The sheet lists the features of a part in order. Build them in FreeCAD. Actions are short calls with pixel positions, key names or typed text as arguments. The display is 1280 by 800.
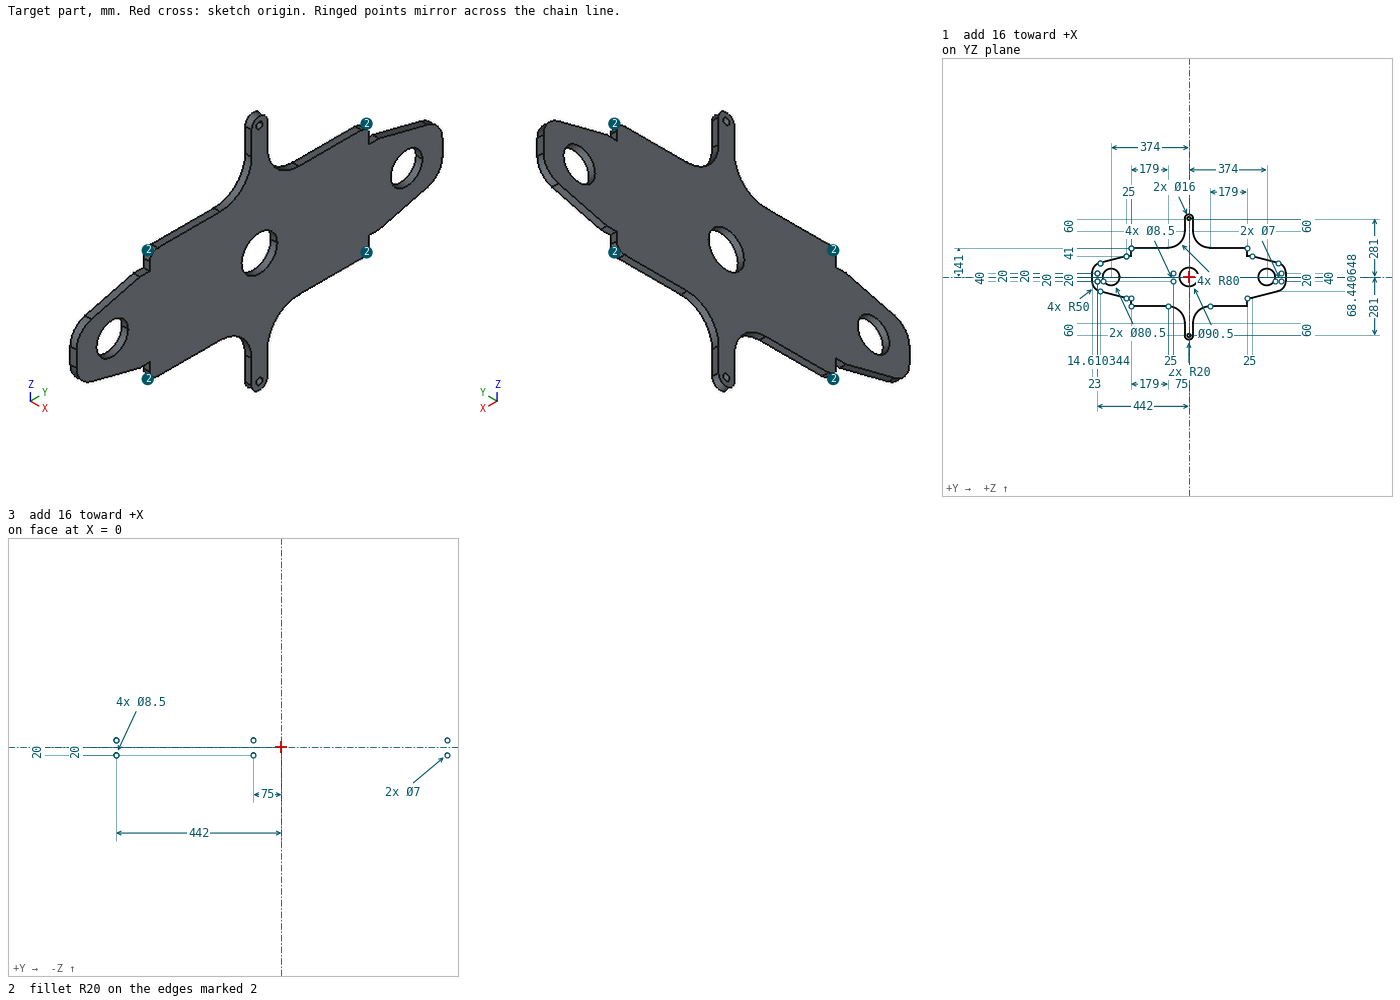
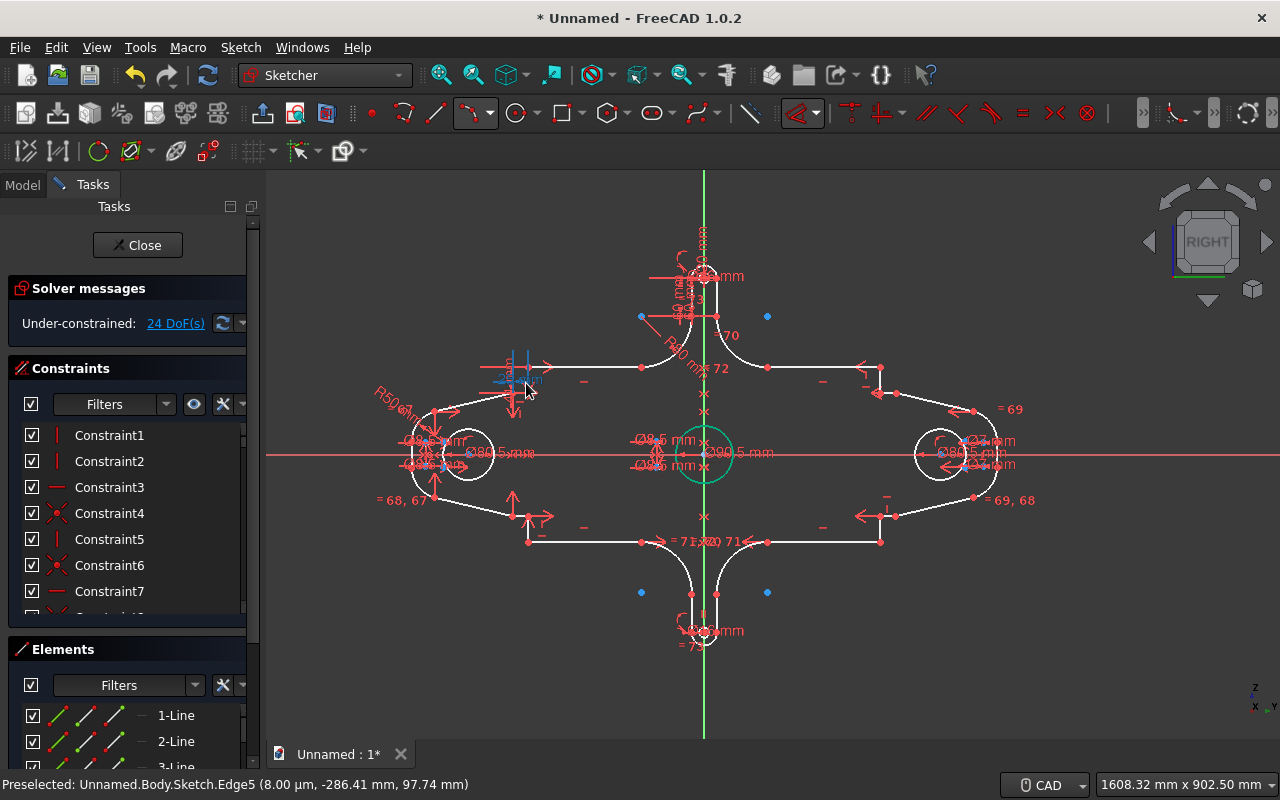
scroll(412, 450, up, 6)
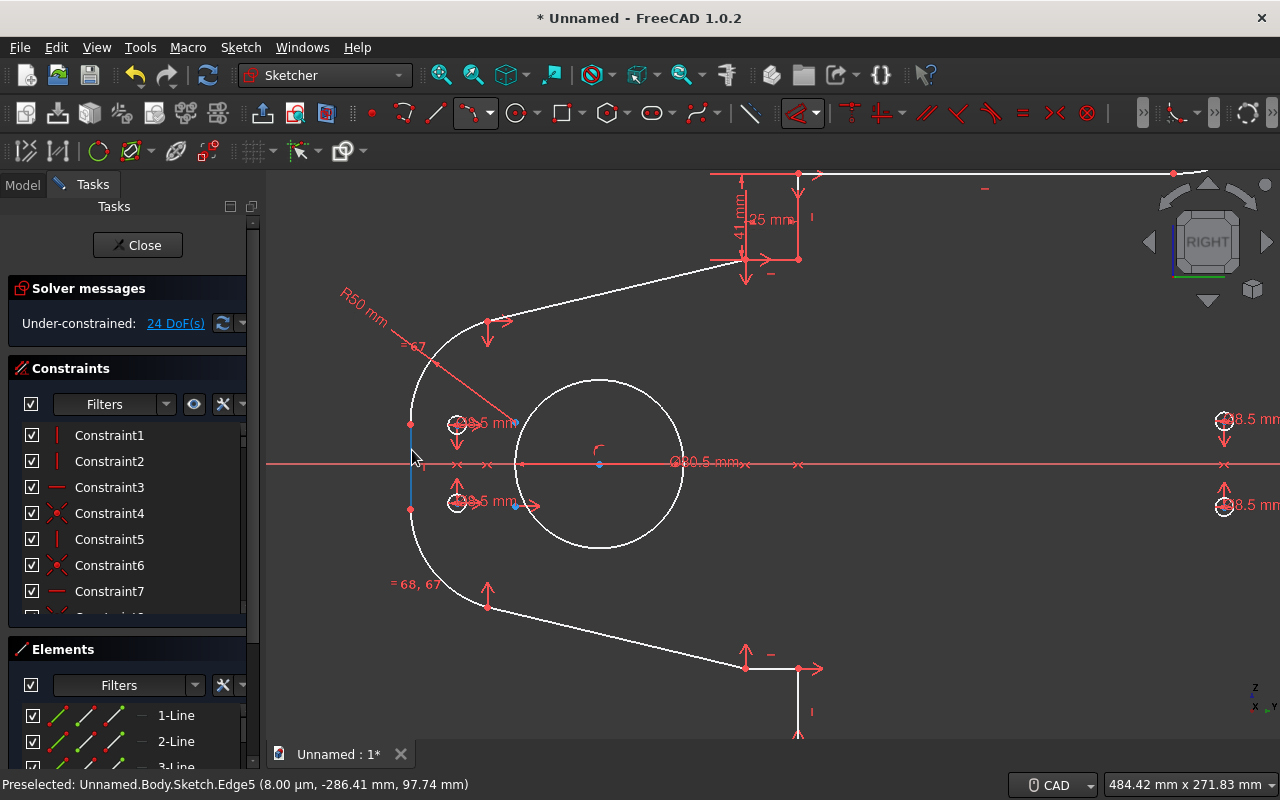
click(411, 450)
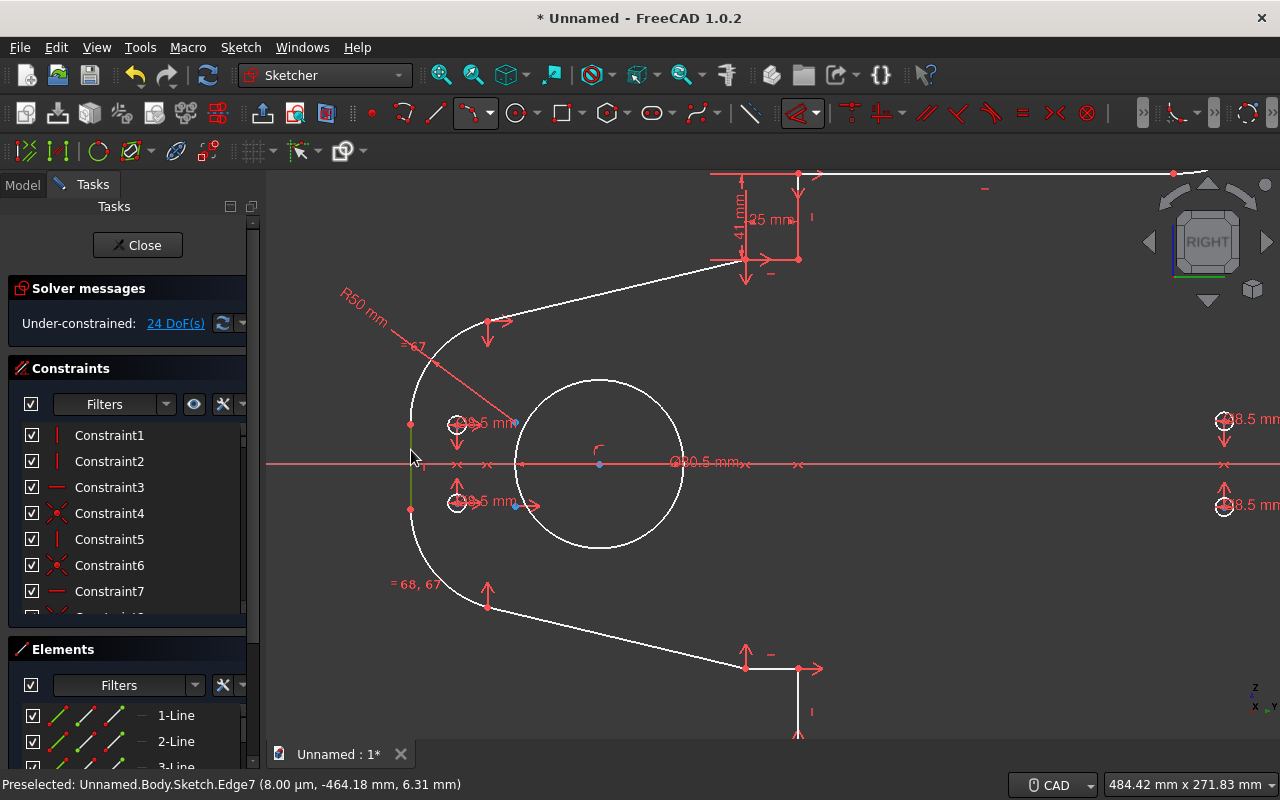
key(i)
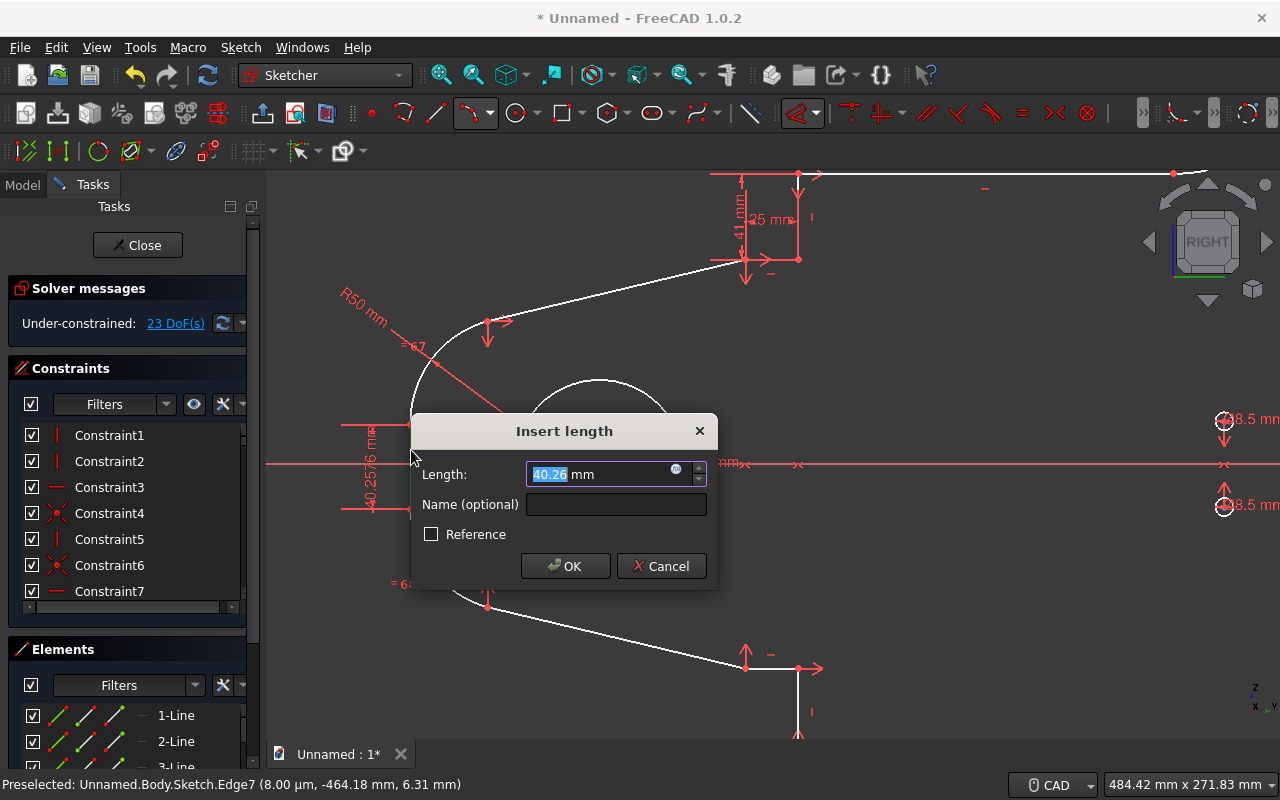
text(40)
key(Return)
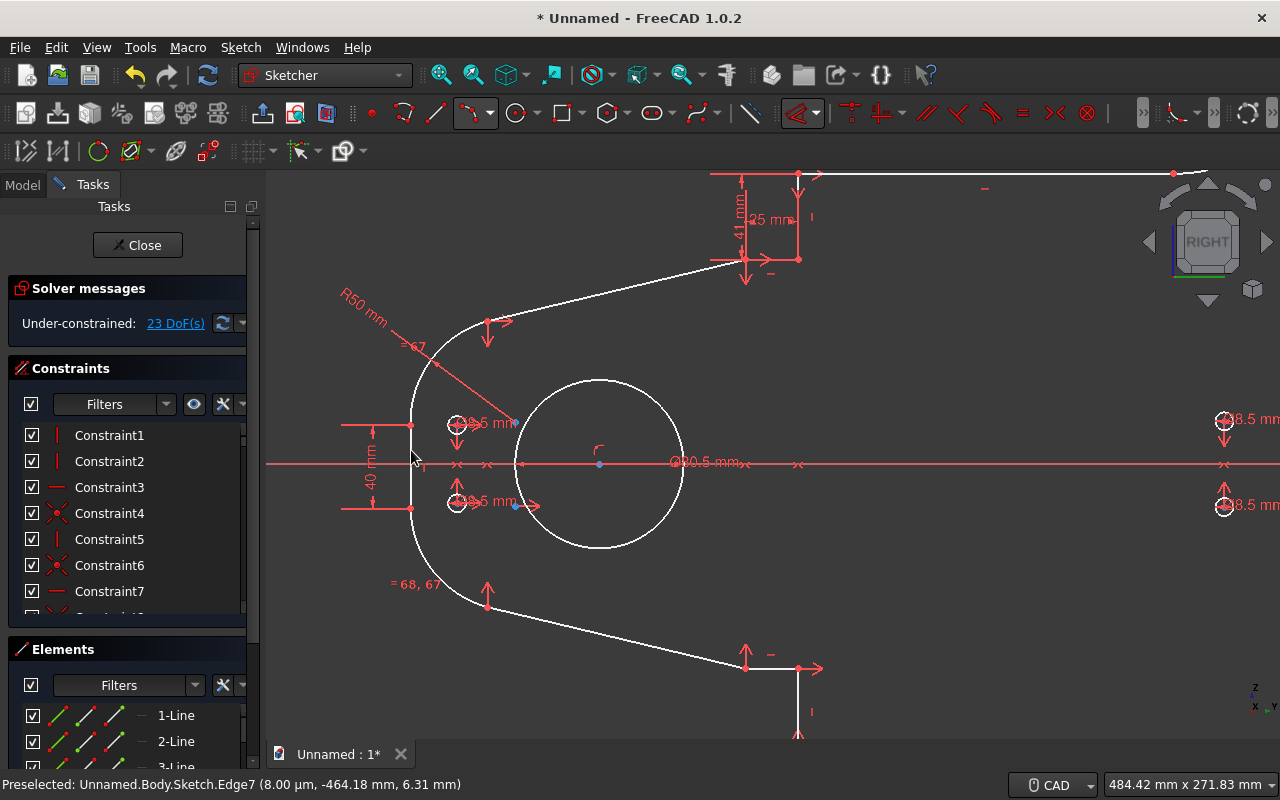
scroll(412, 450, down, 6)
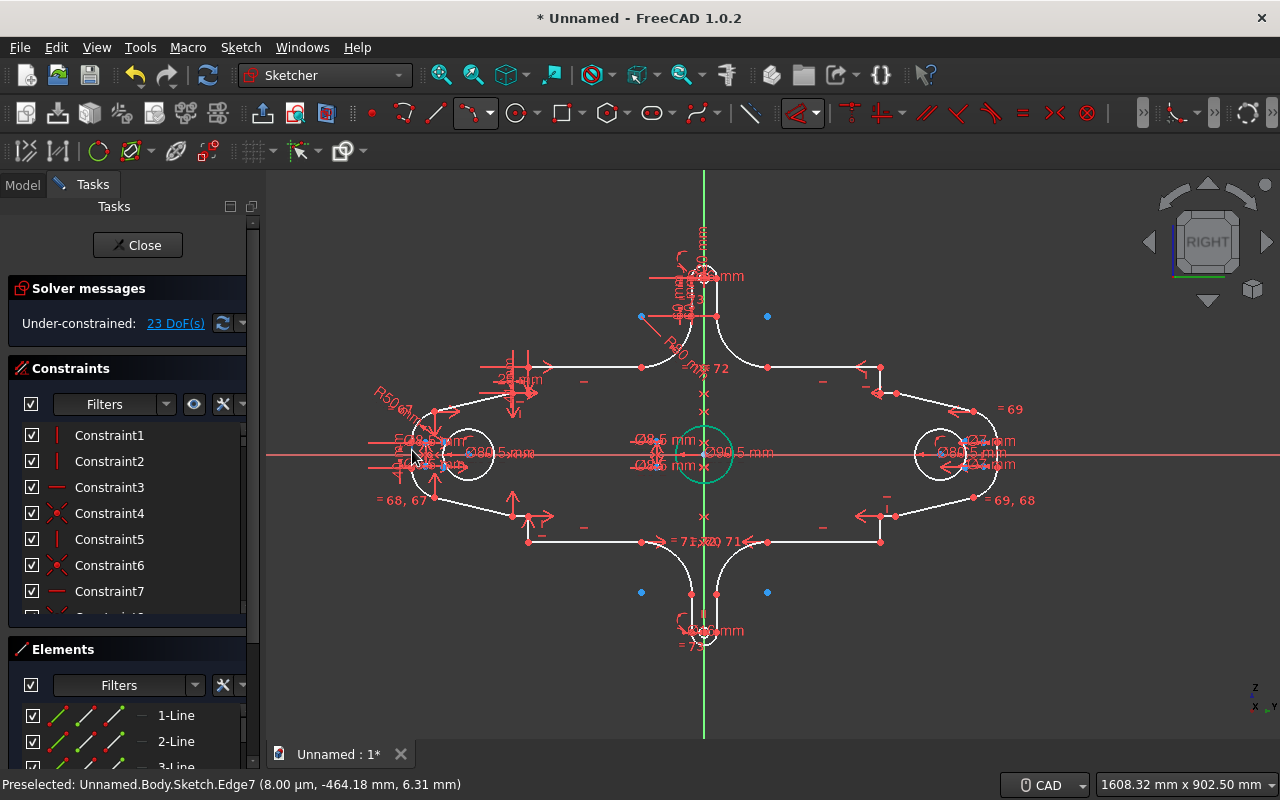
click(692, 606)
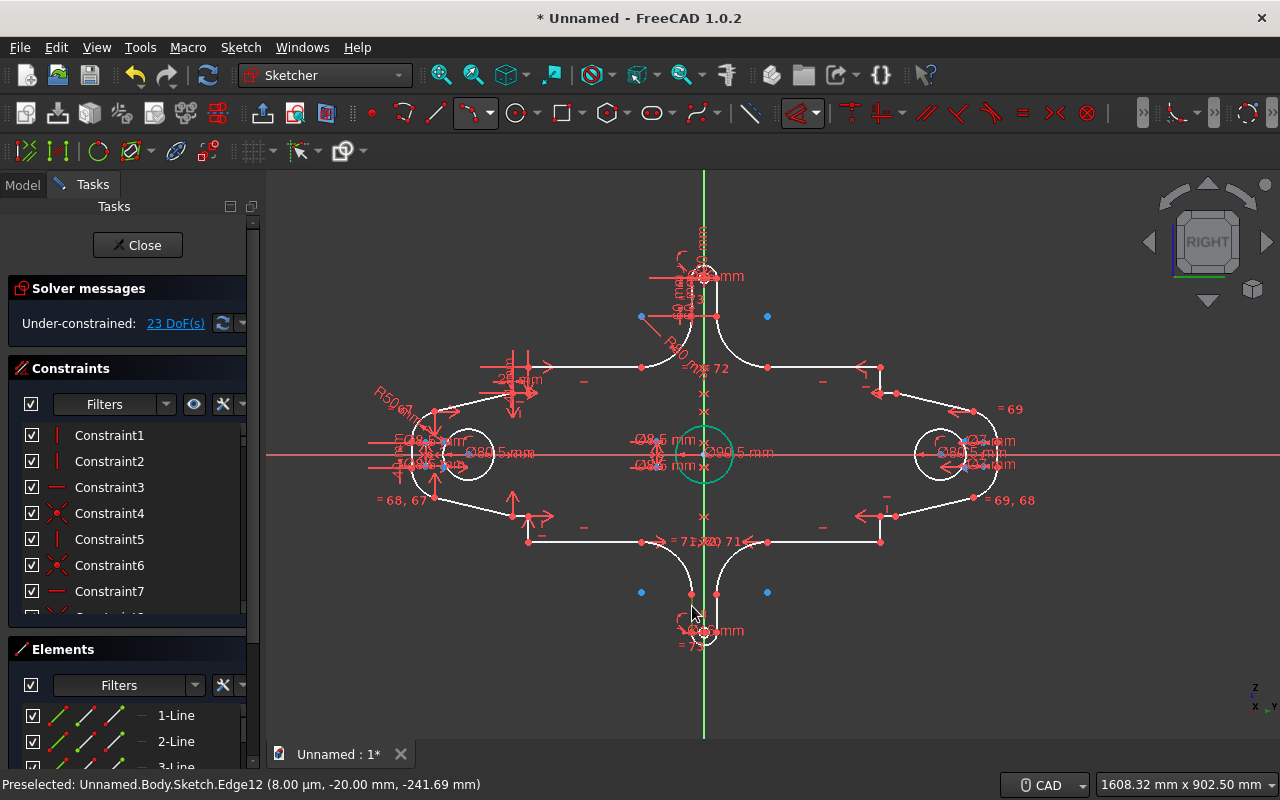
key(i)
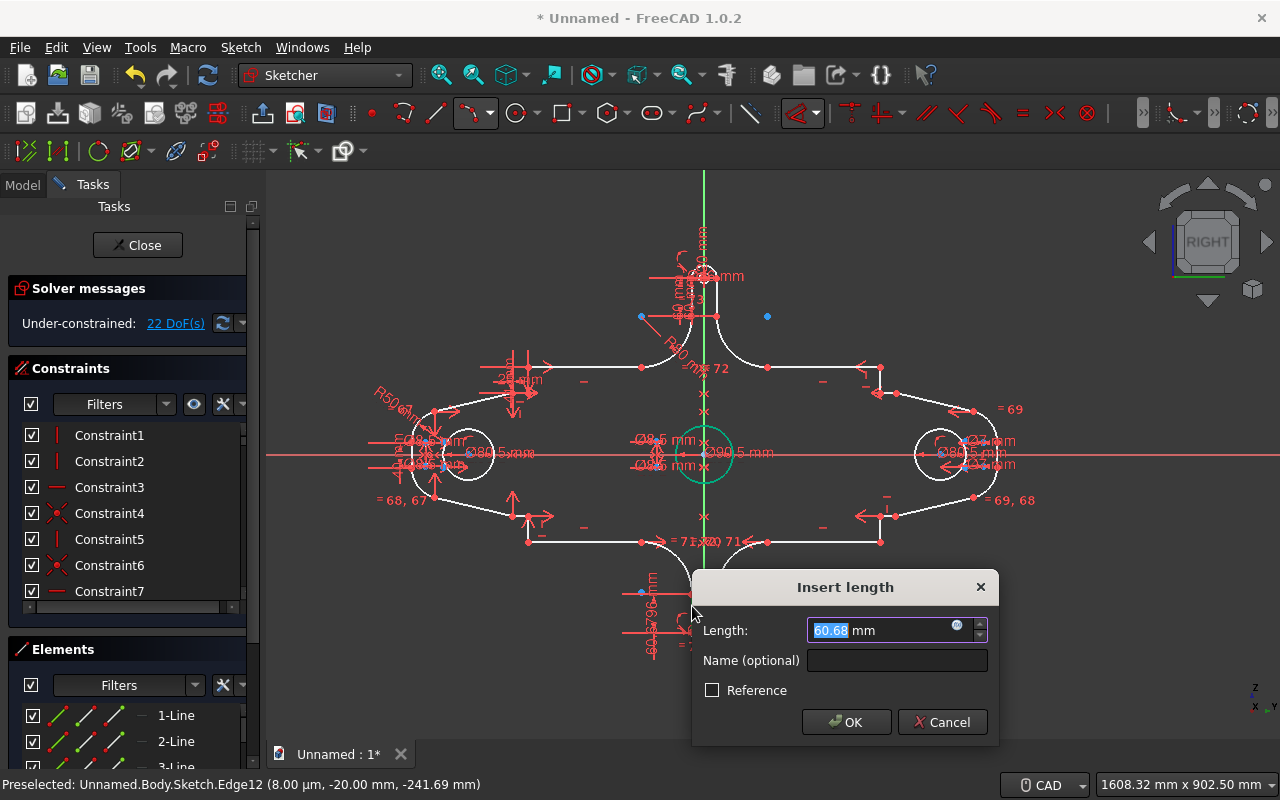
text(60)
key(Return)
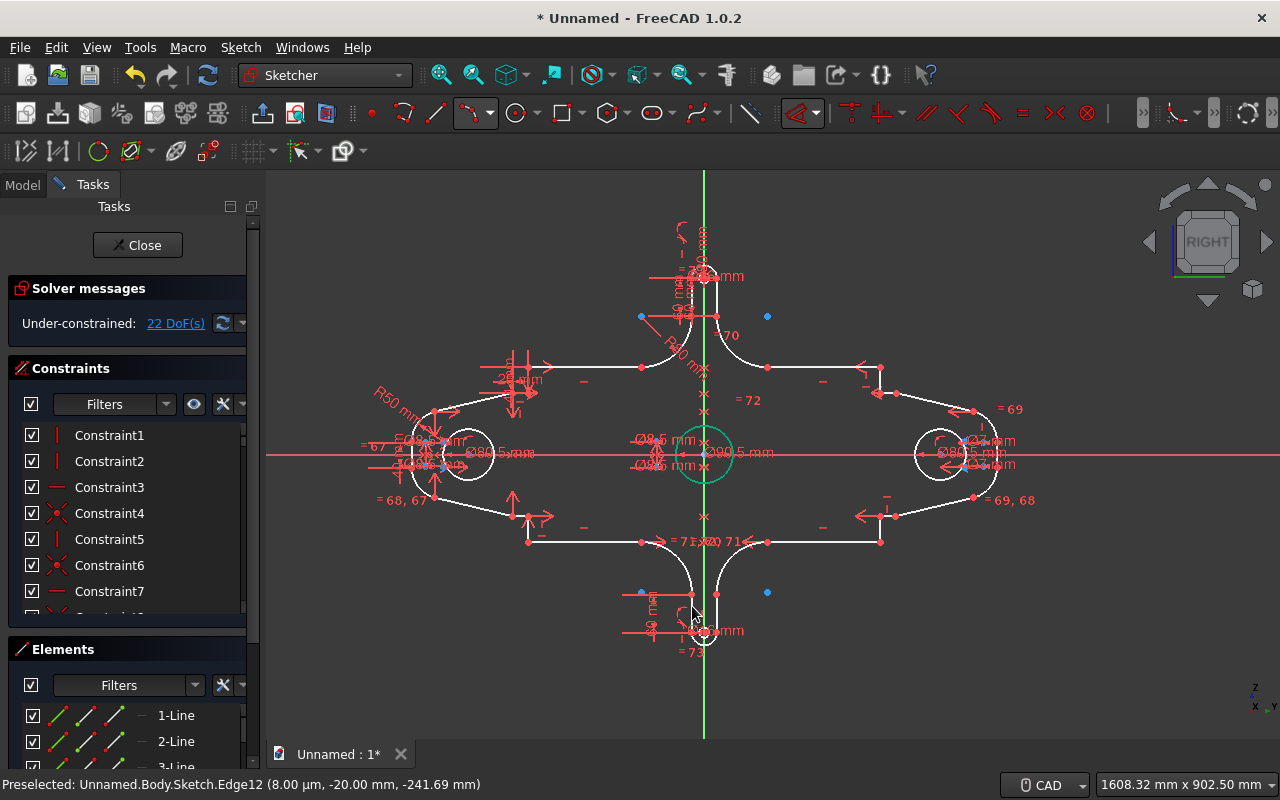
click(717, 621)